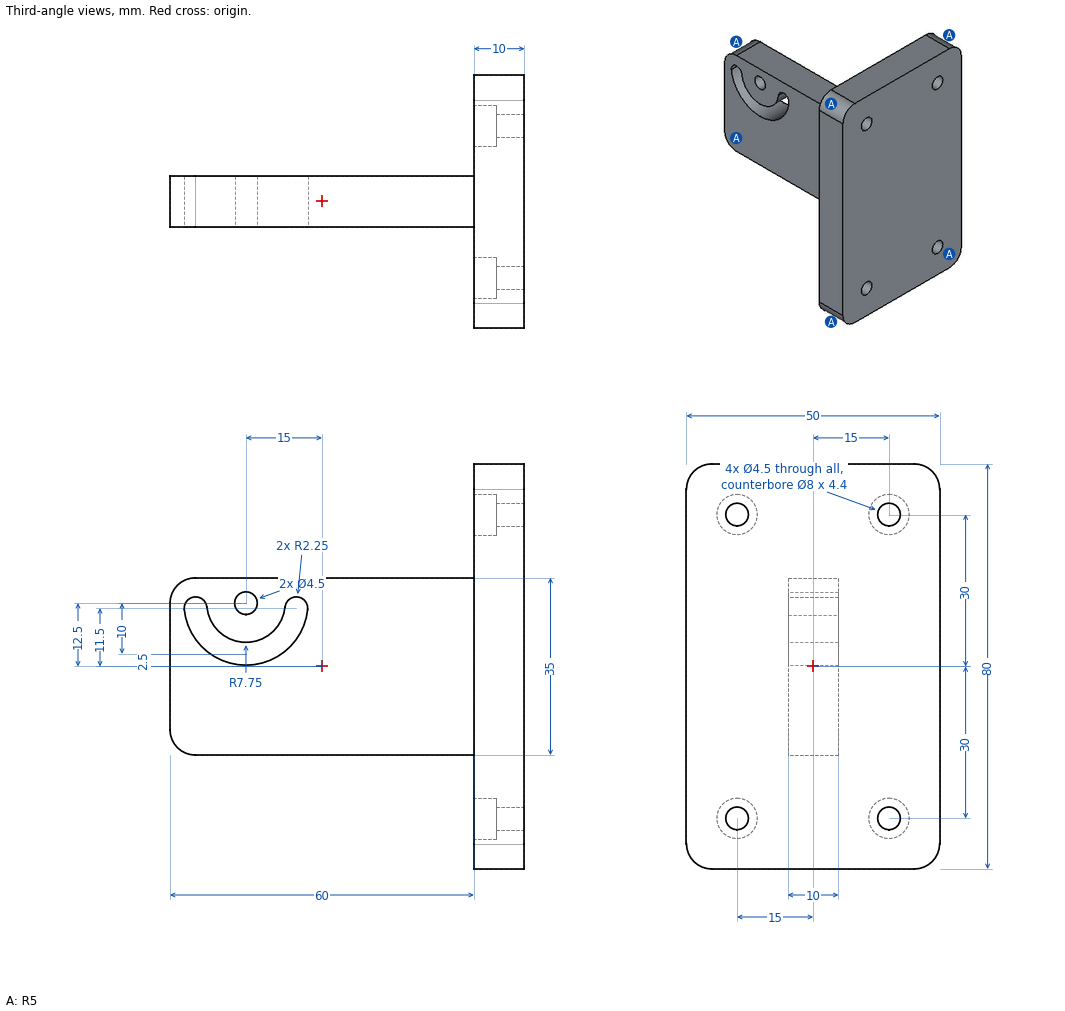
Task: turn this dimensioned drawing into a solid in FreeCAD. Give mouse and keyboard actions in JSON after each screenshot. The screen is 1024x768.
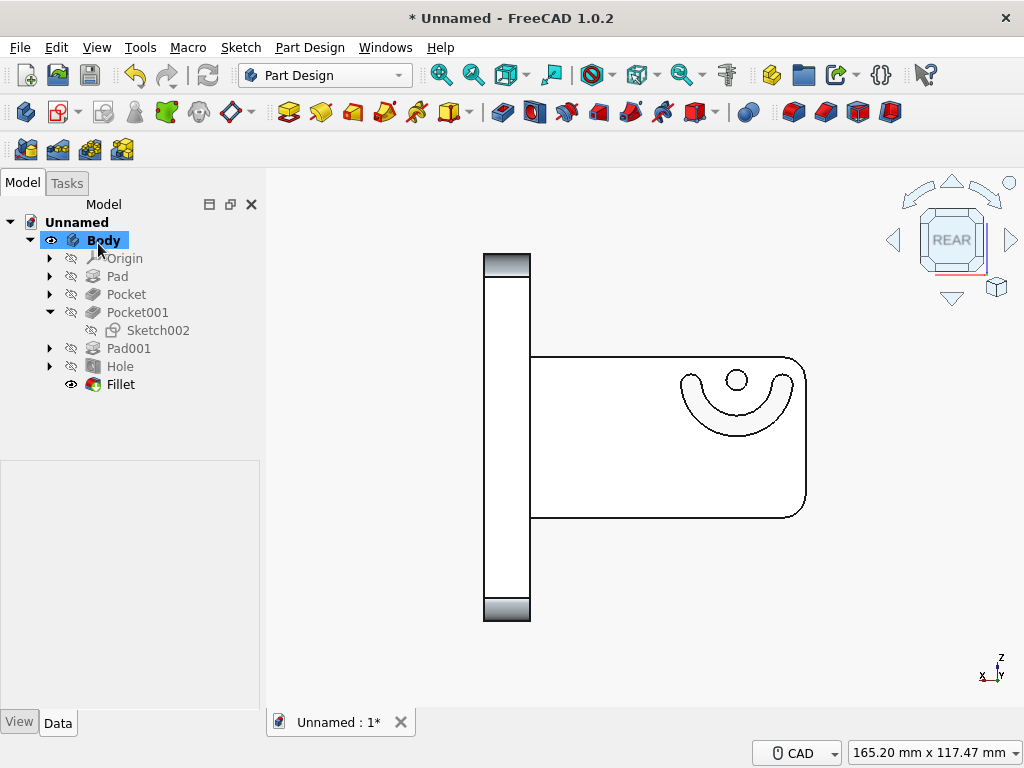
{"action": "key", "text": "0"}